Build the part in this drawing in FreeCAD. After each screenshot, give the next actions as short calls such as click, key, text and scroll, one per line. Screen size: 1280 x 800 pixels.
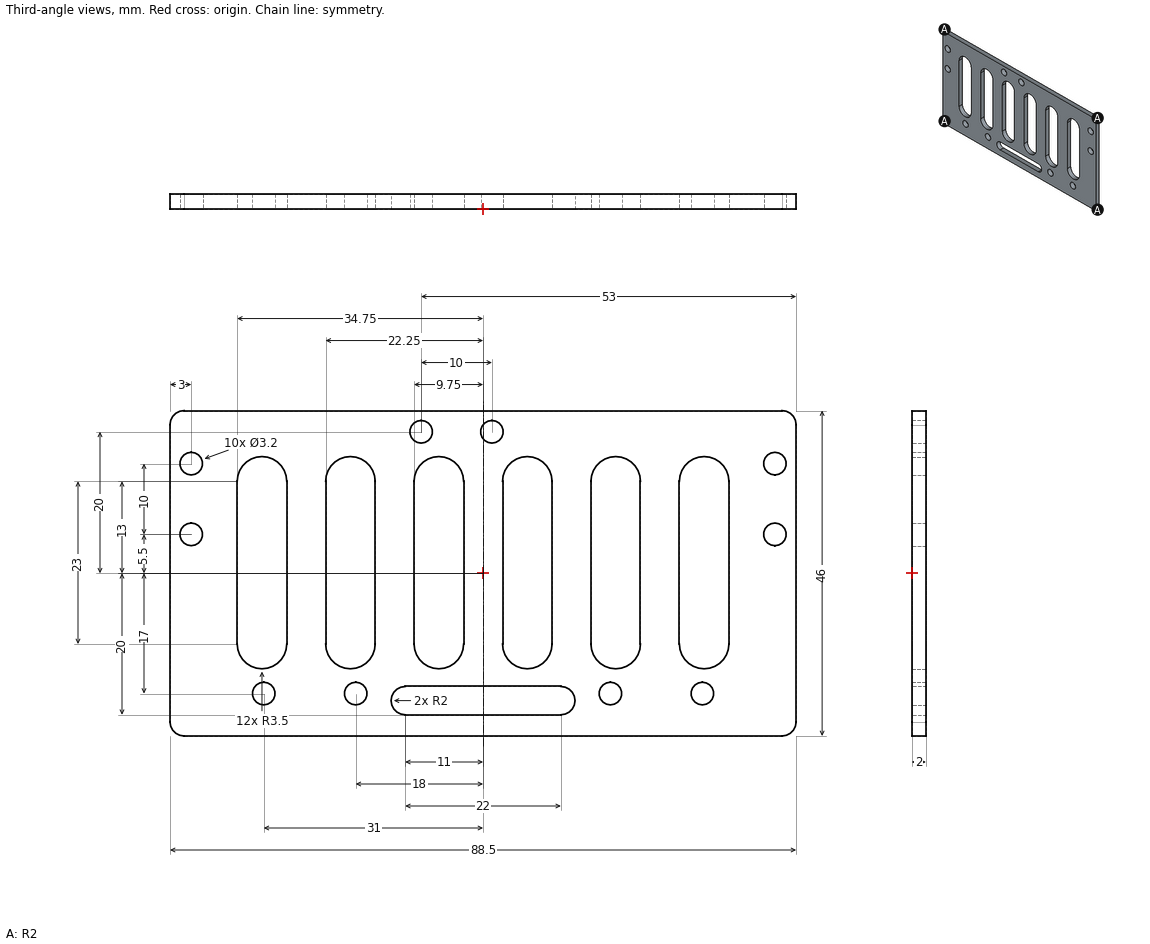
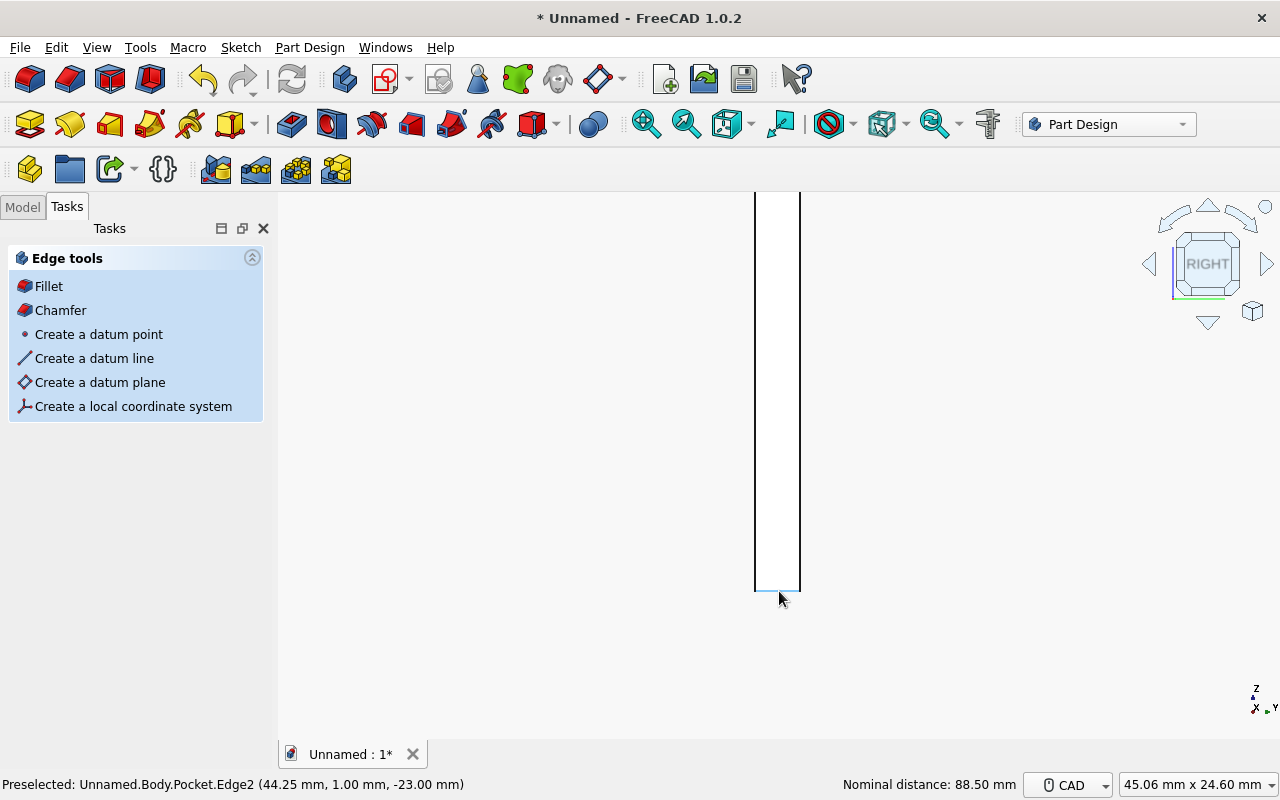
click(777, 590, ctrl)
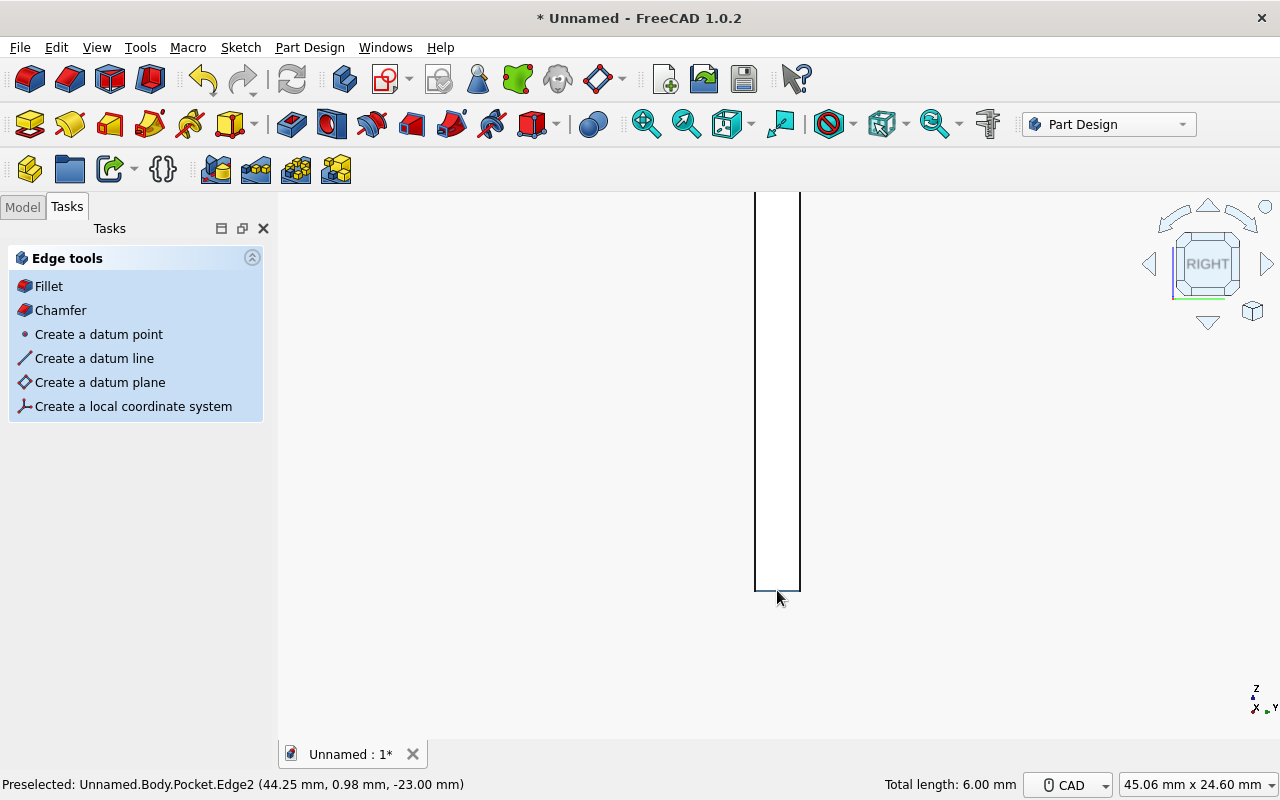
click(648, 124)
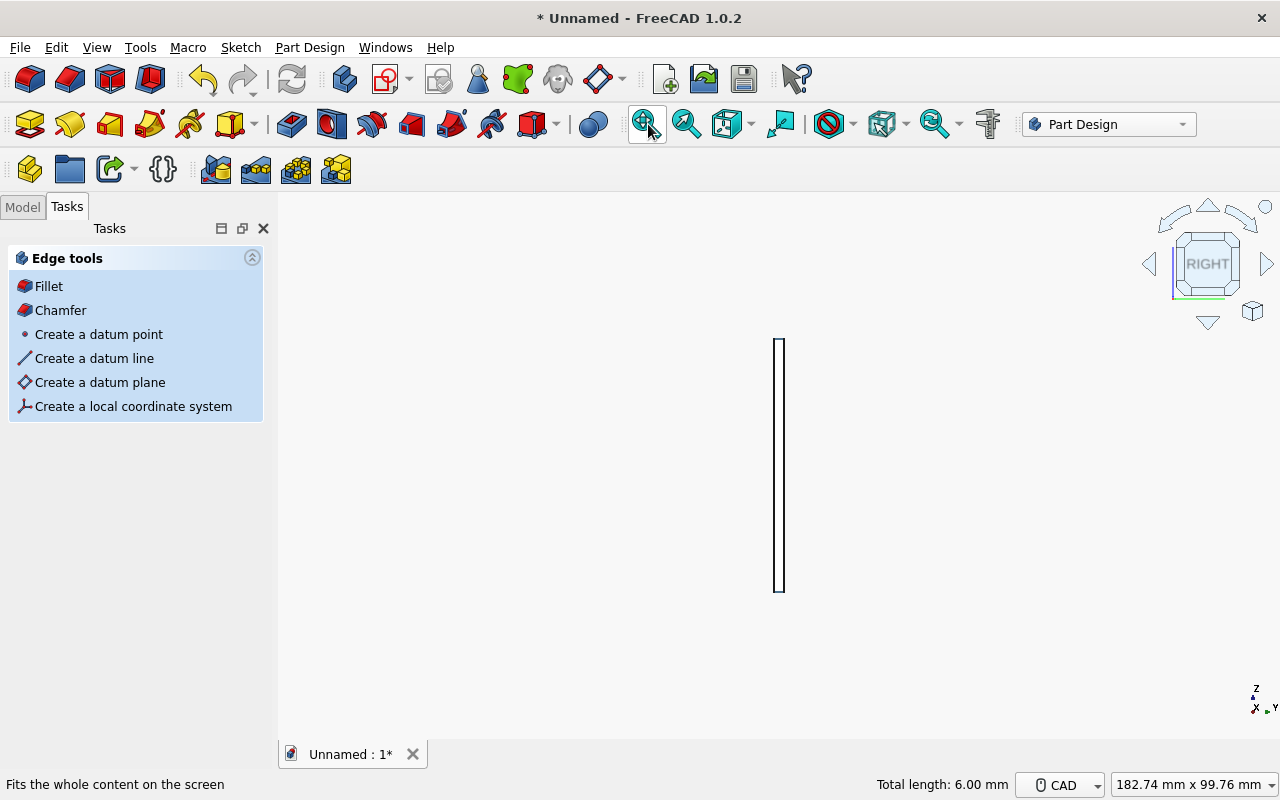
key(5)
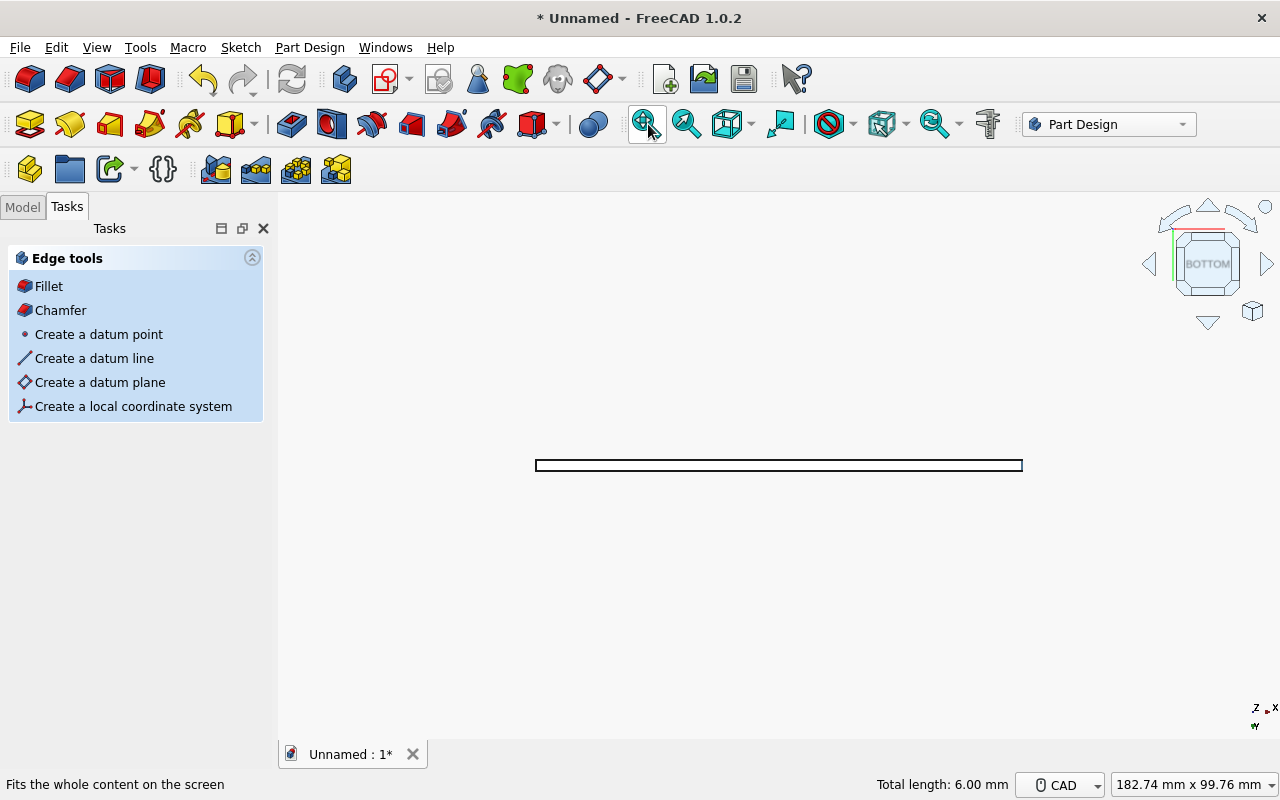
click(536, 466, ctrl)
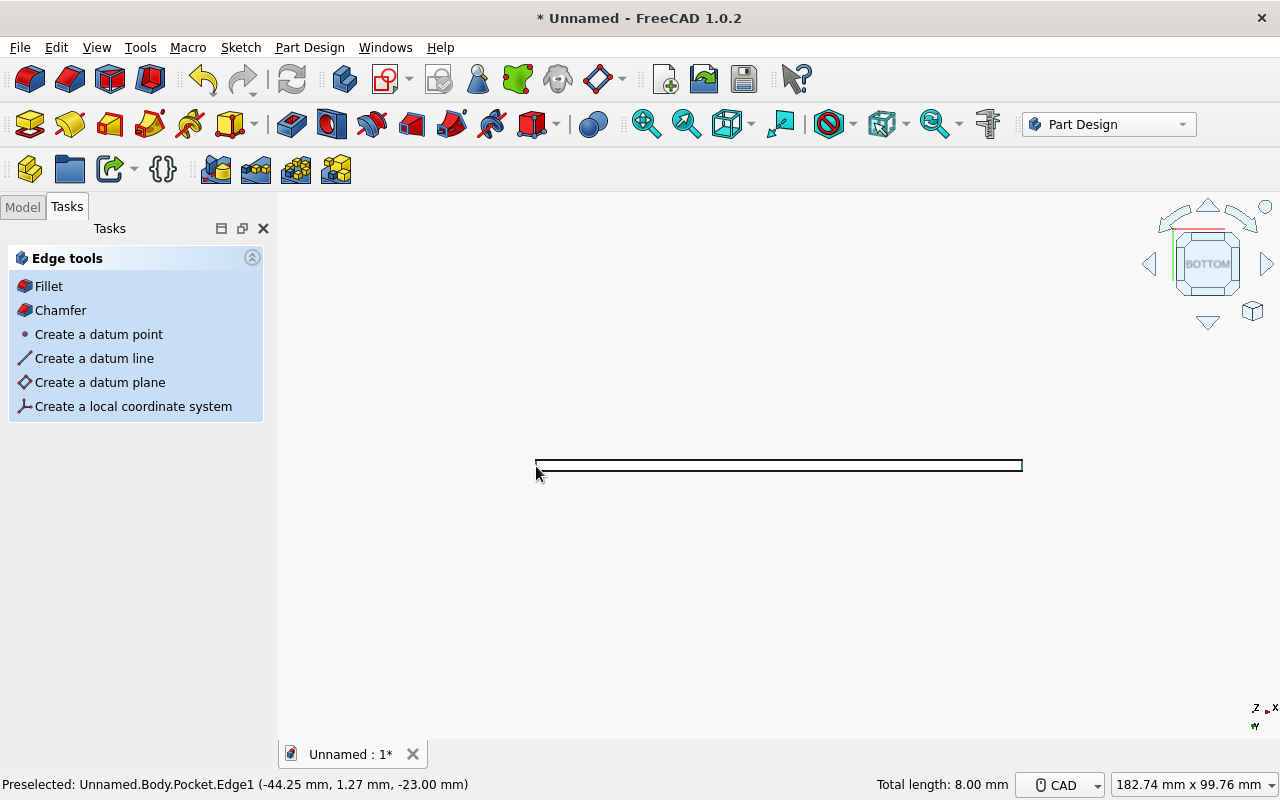
click(30, 80)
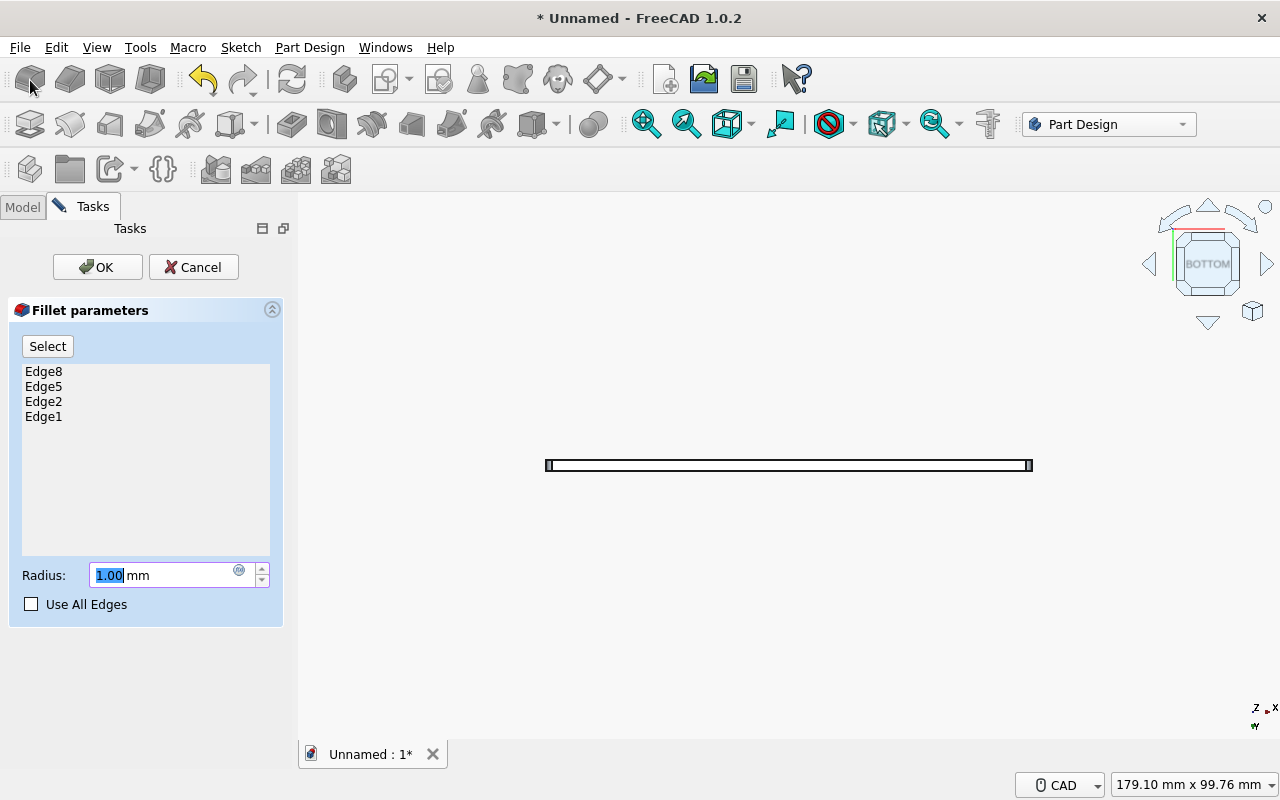
text(2)
key(Tab)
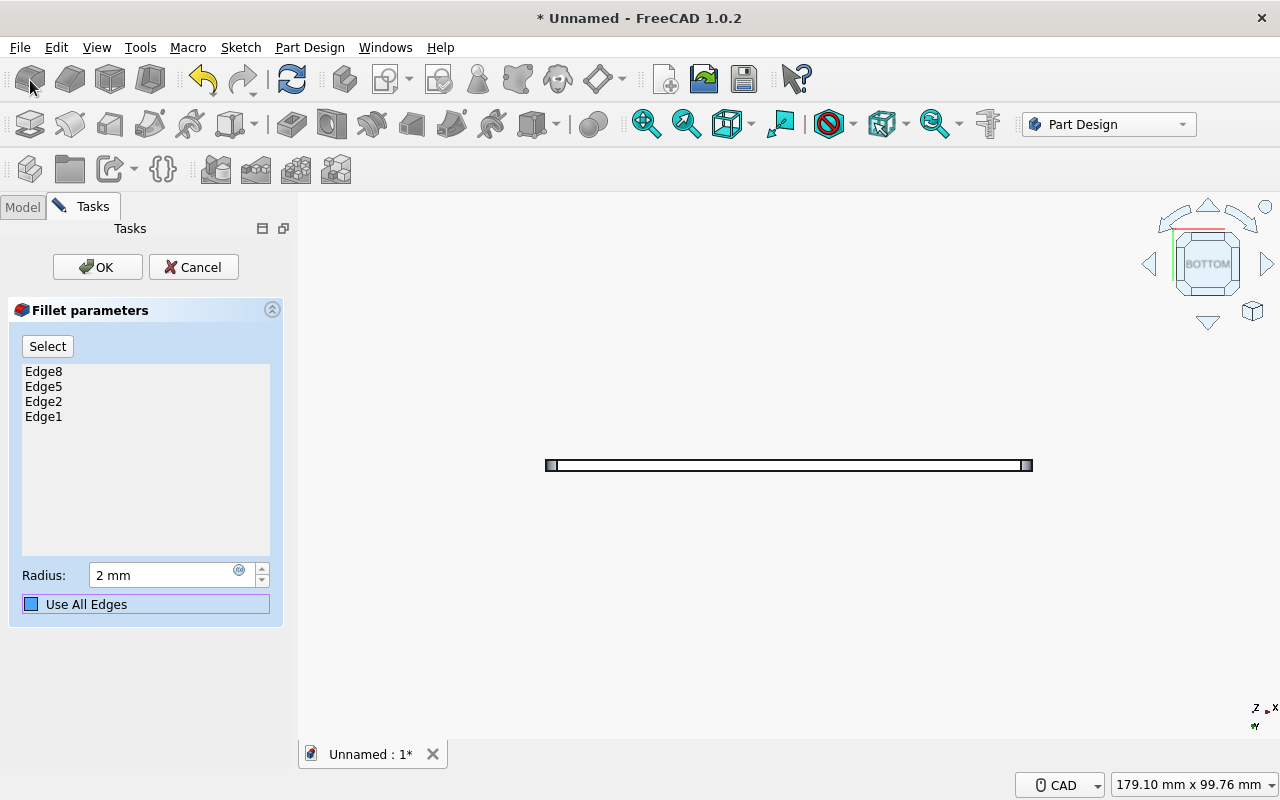
click(98, 267)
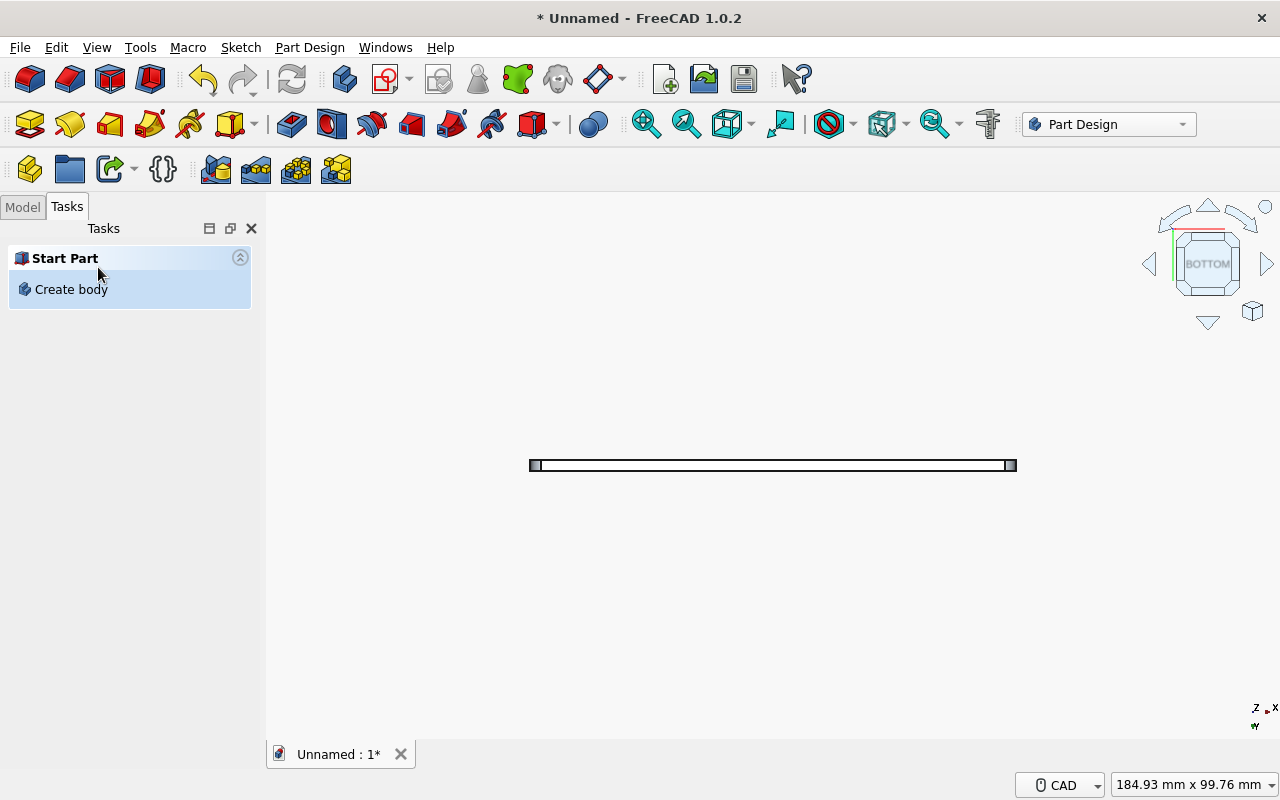
key(0)